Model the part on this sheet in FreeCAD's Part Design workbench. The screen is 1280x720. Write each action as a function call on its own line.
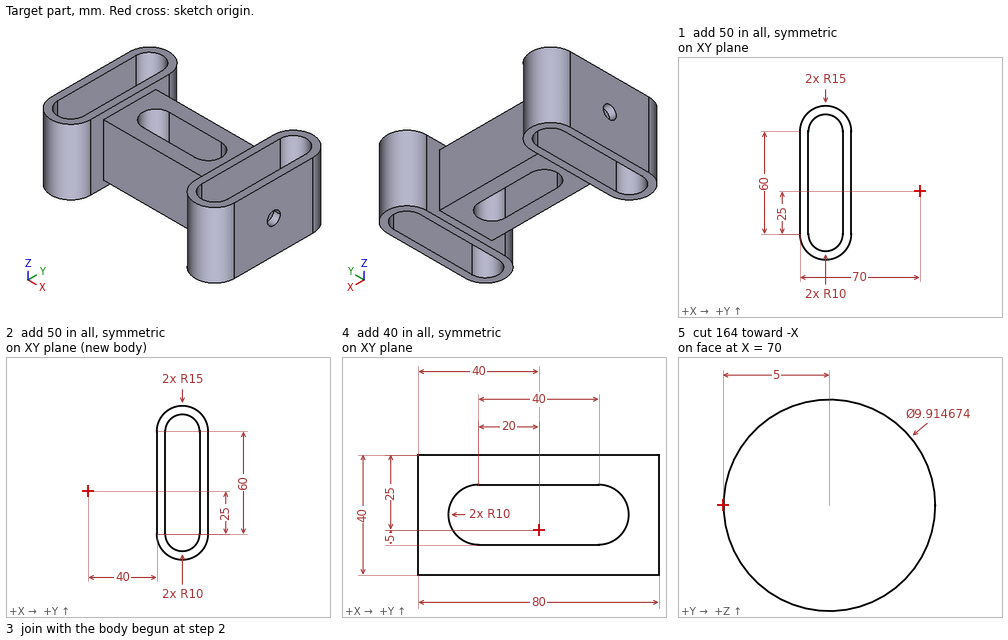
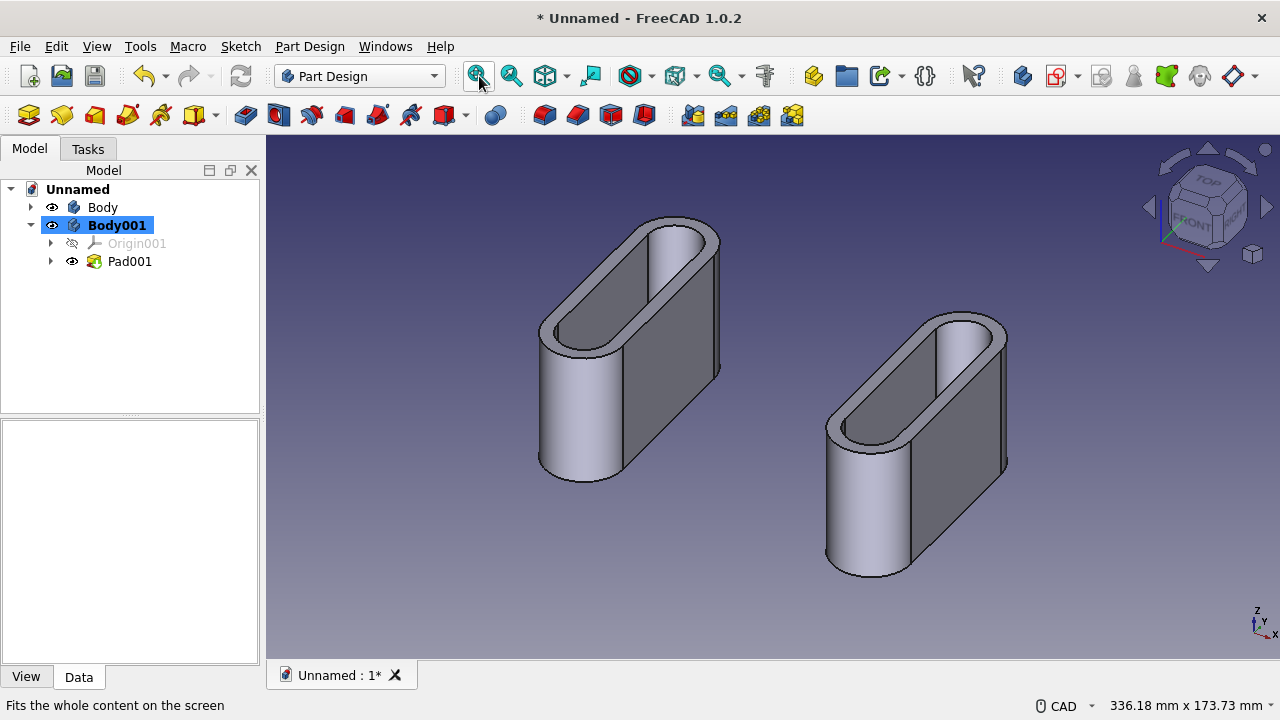
double_click(97, 207)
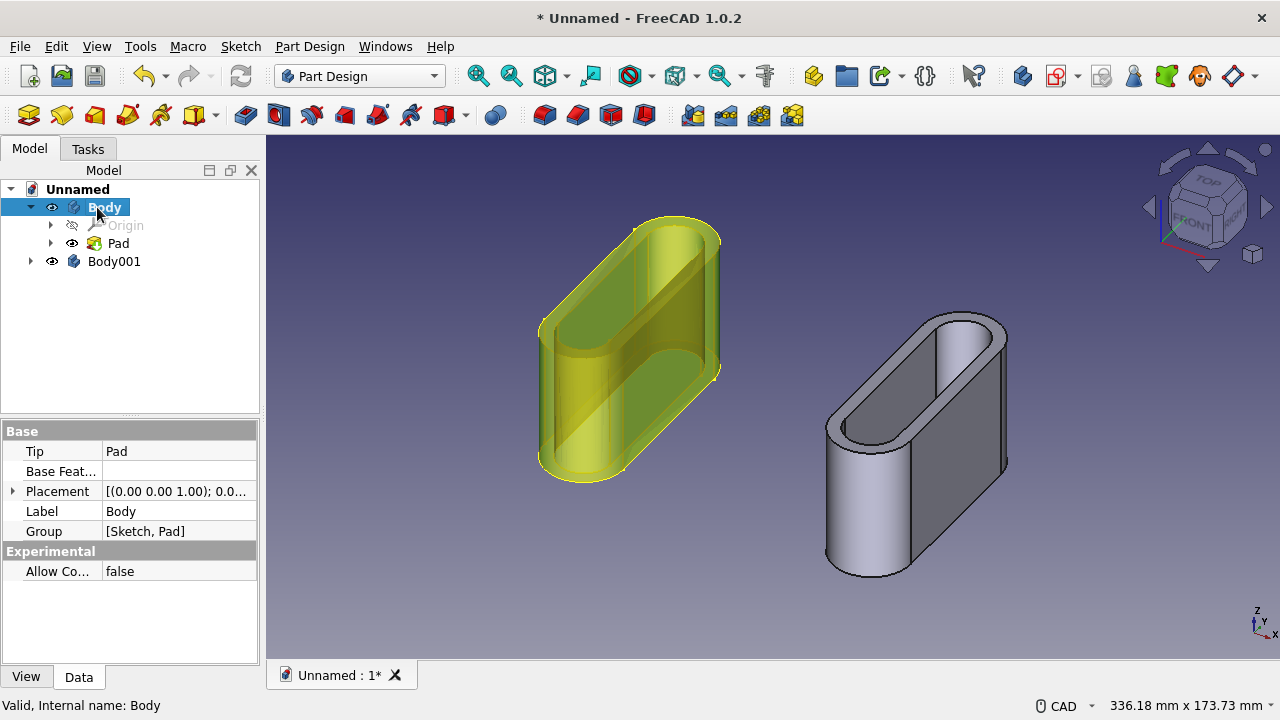
click(97, 207)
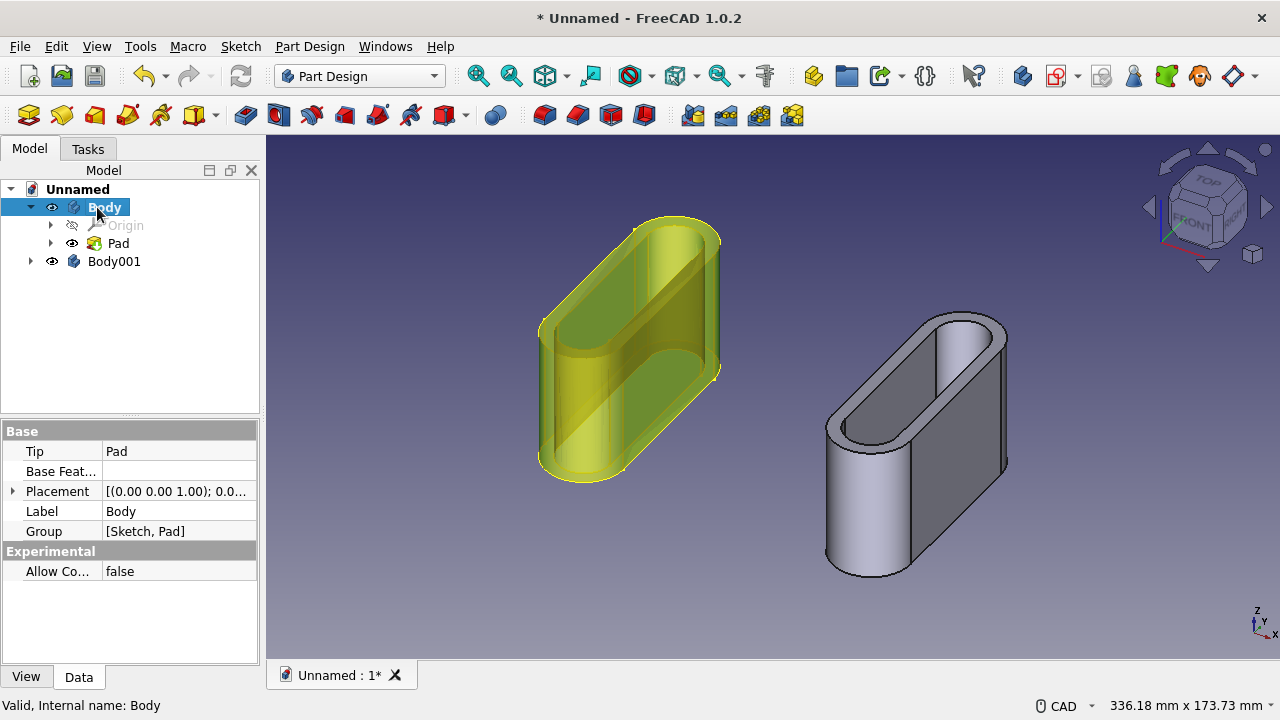
click(148, 571)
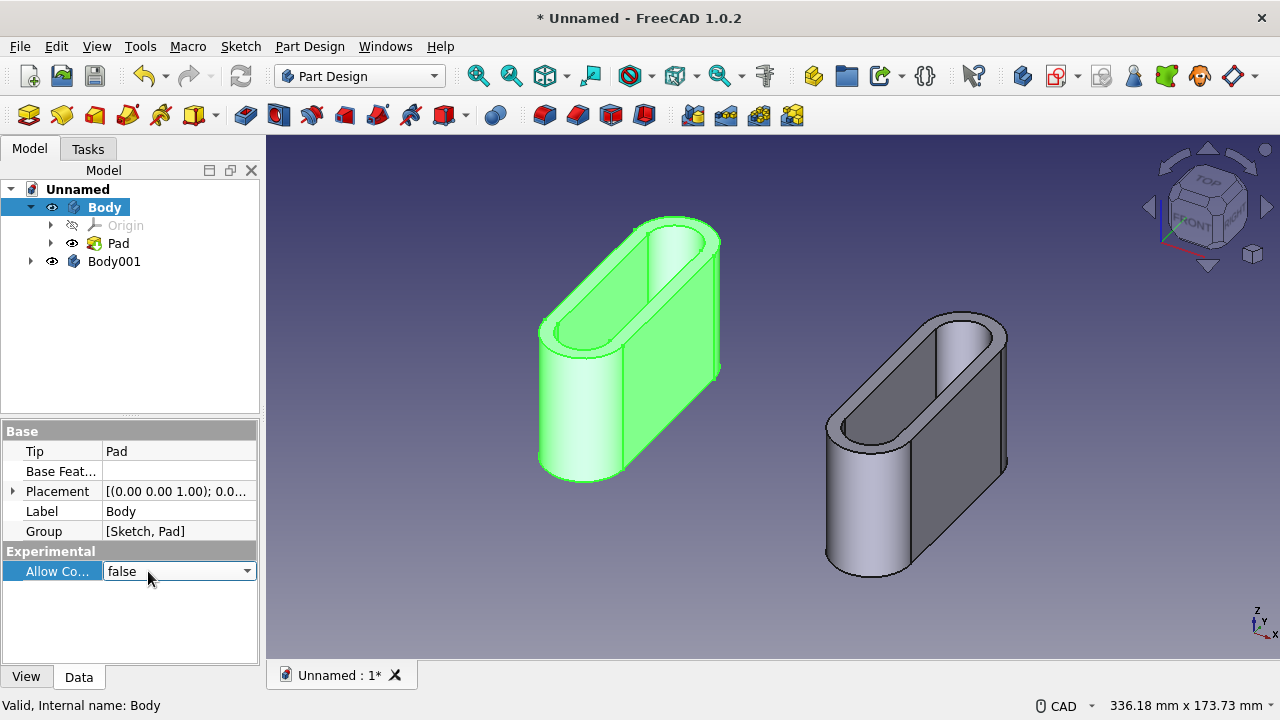
click(148, 571)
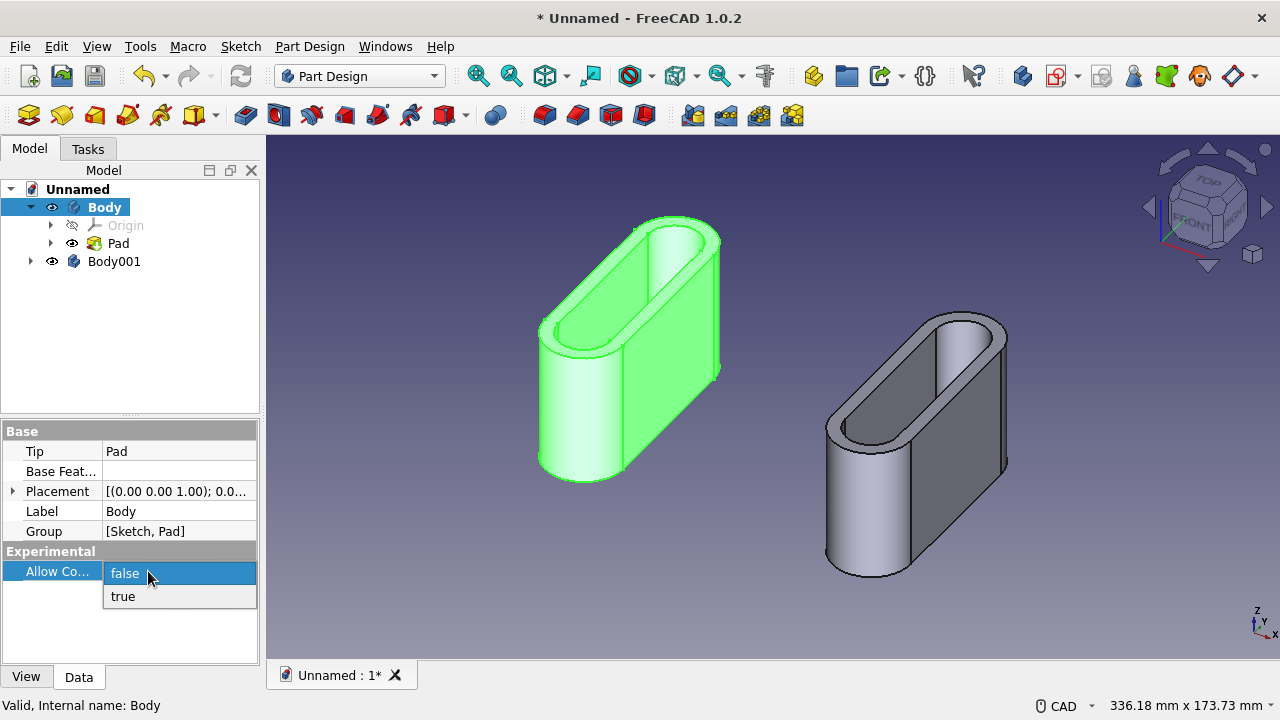
click(178, 596)
key(Return)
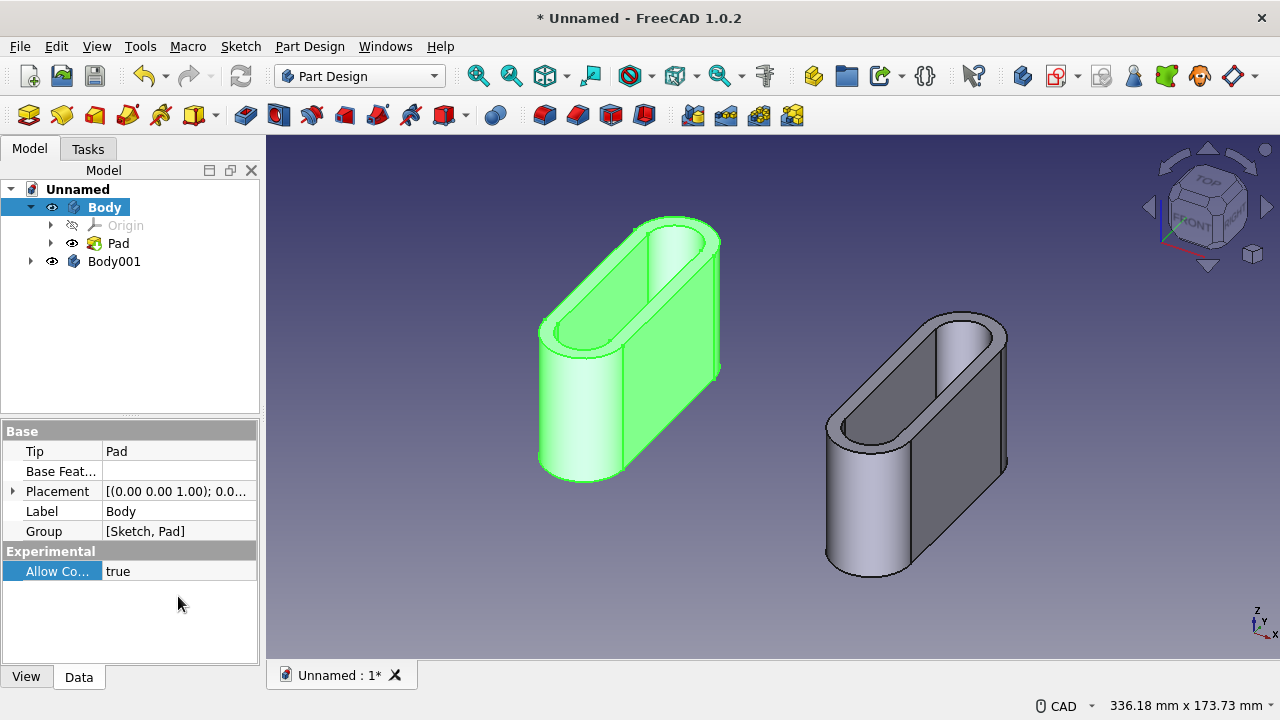
click(97, 261)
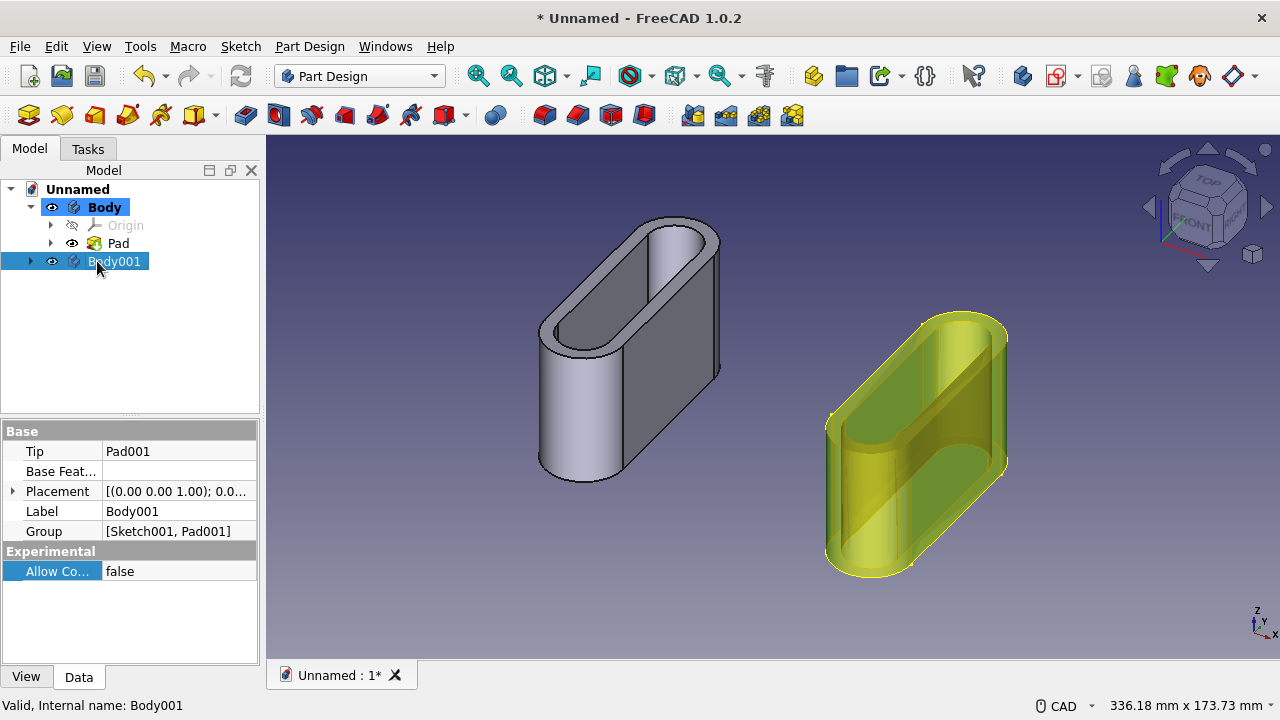
click(496, 116)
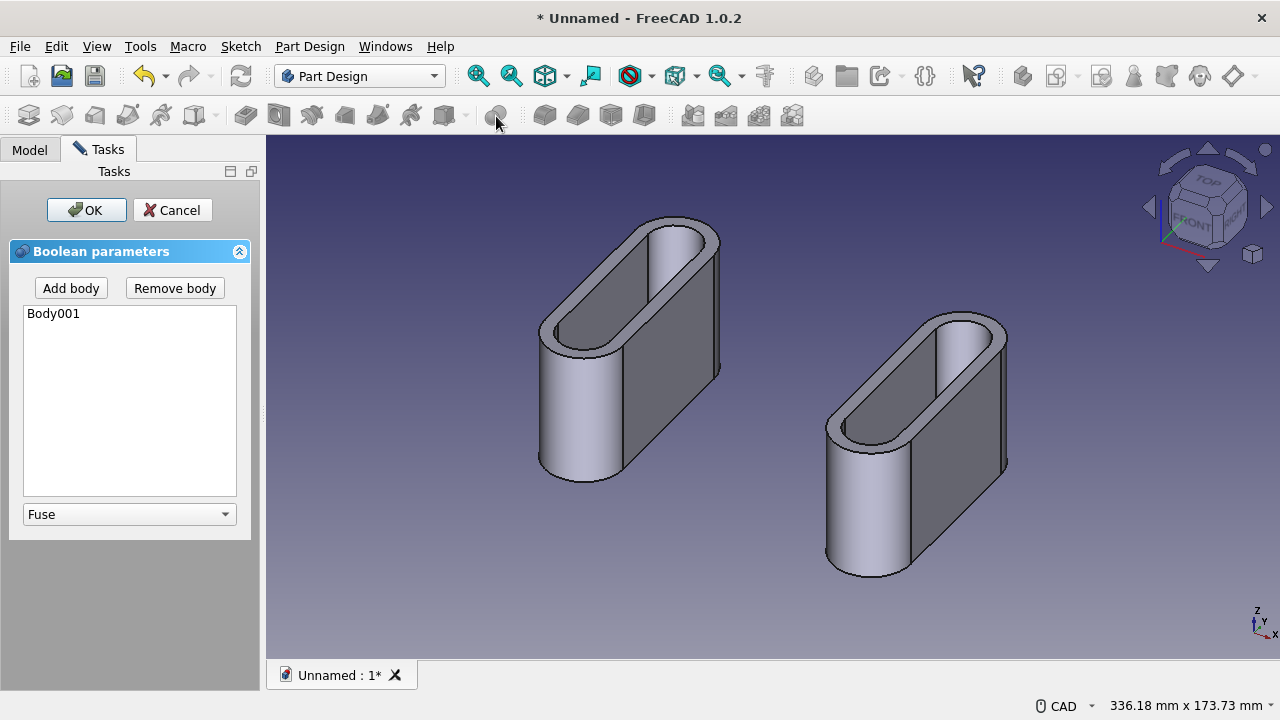
click(87, 210)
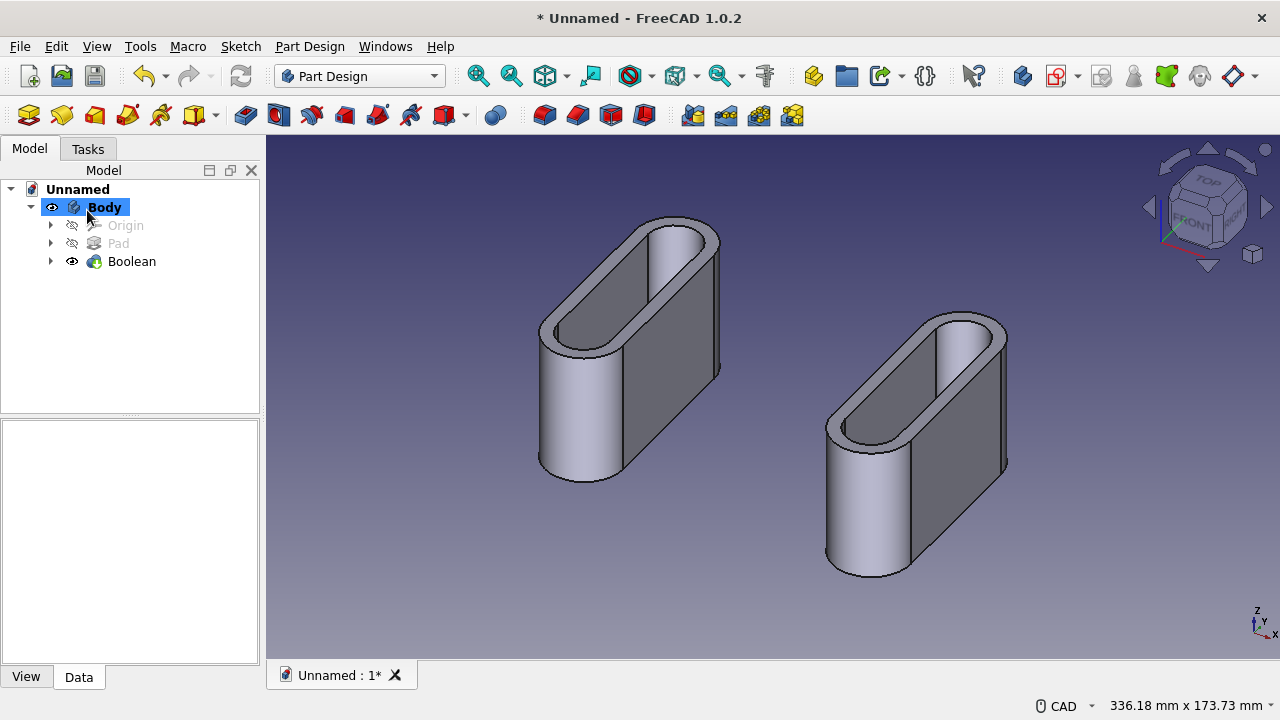
click(1056, 76)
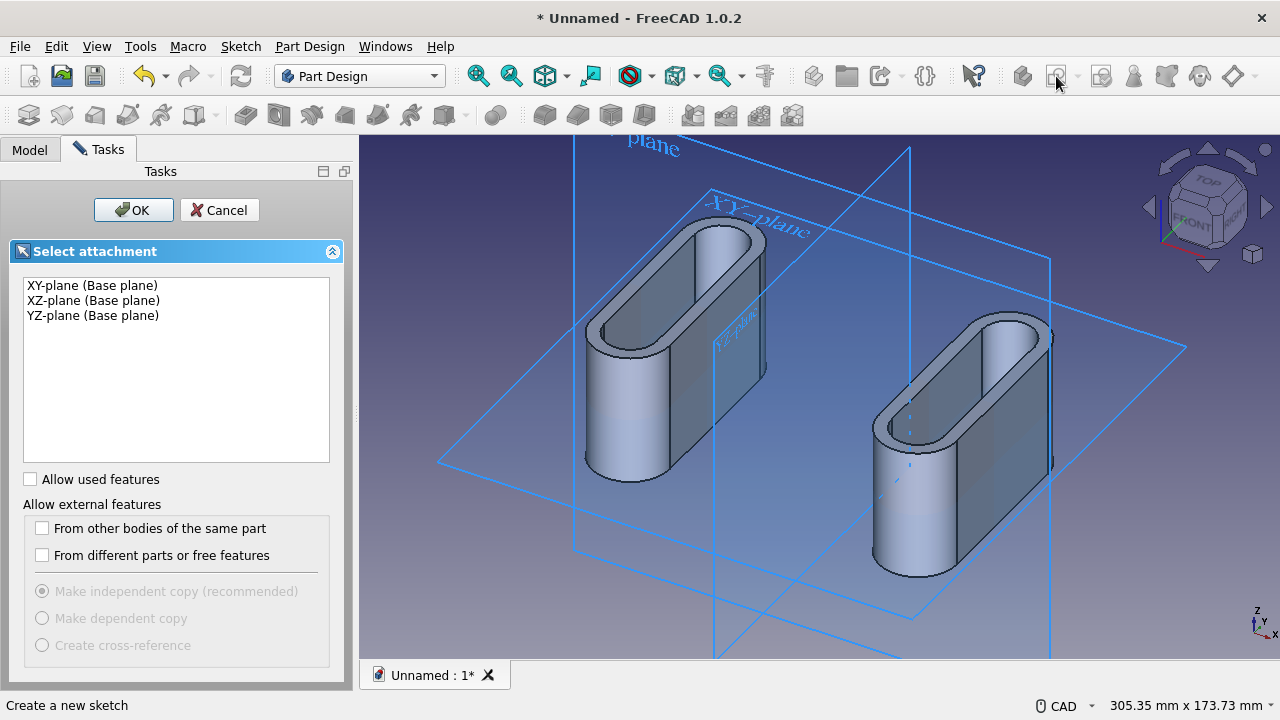
click(84, 286)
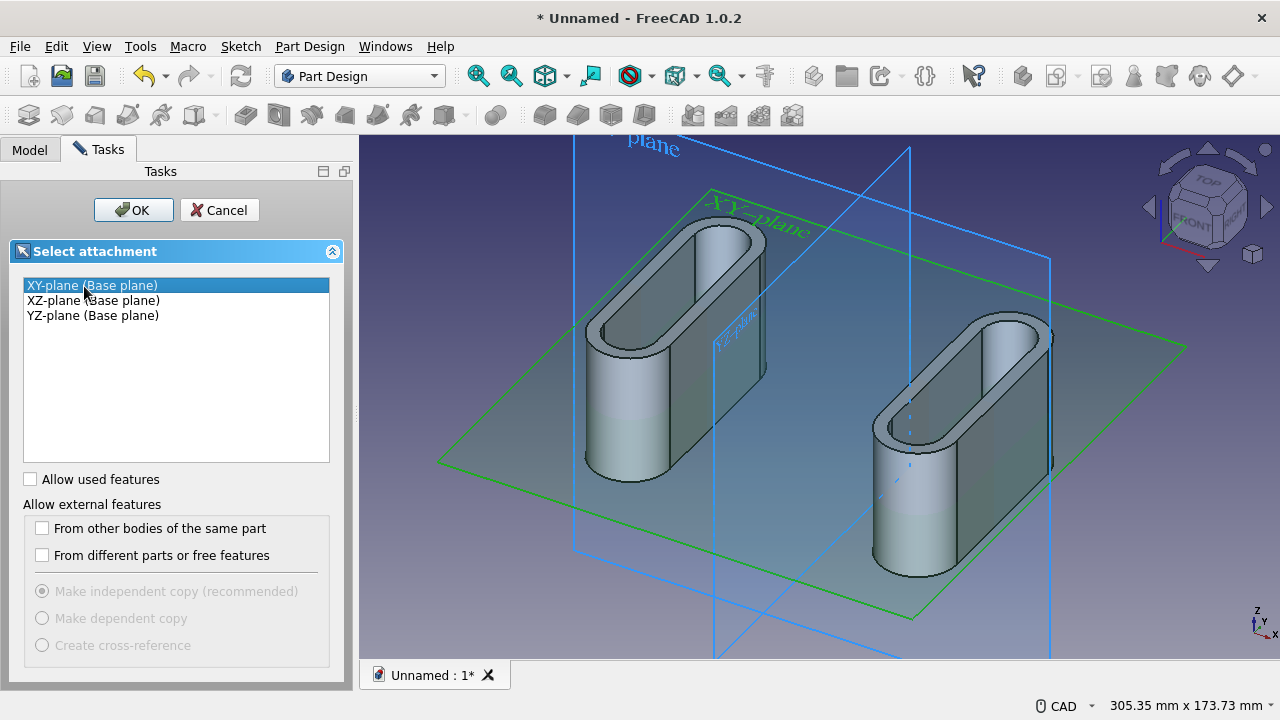
click(134, 210)